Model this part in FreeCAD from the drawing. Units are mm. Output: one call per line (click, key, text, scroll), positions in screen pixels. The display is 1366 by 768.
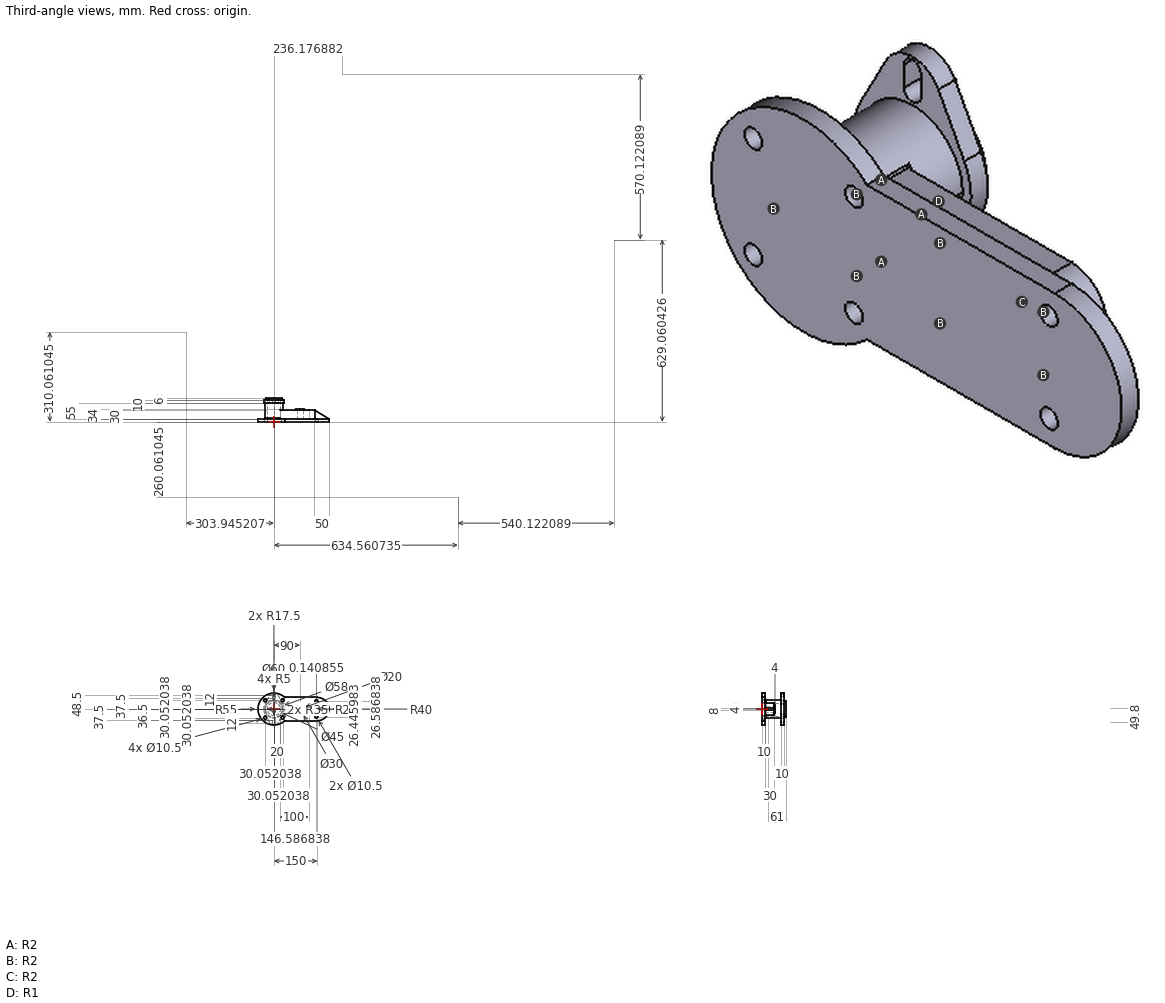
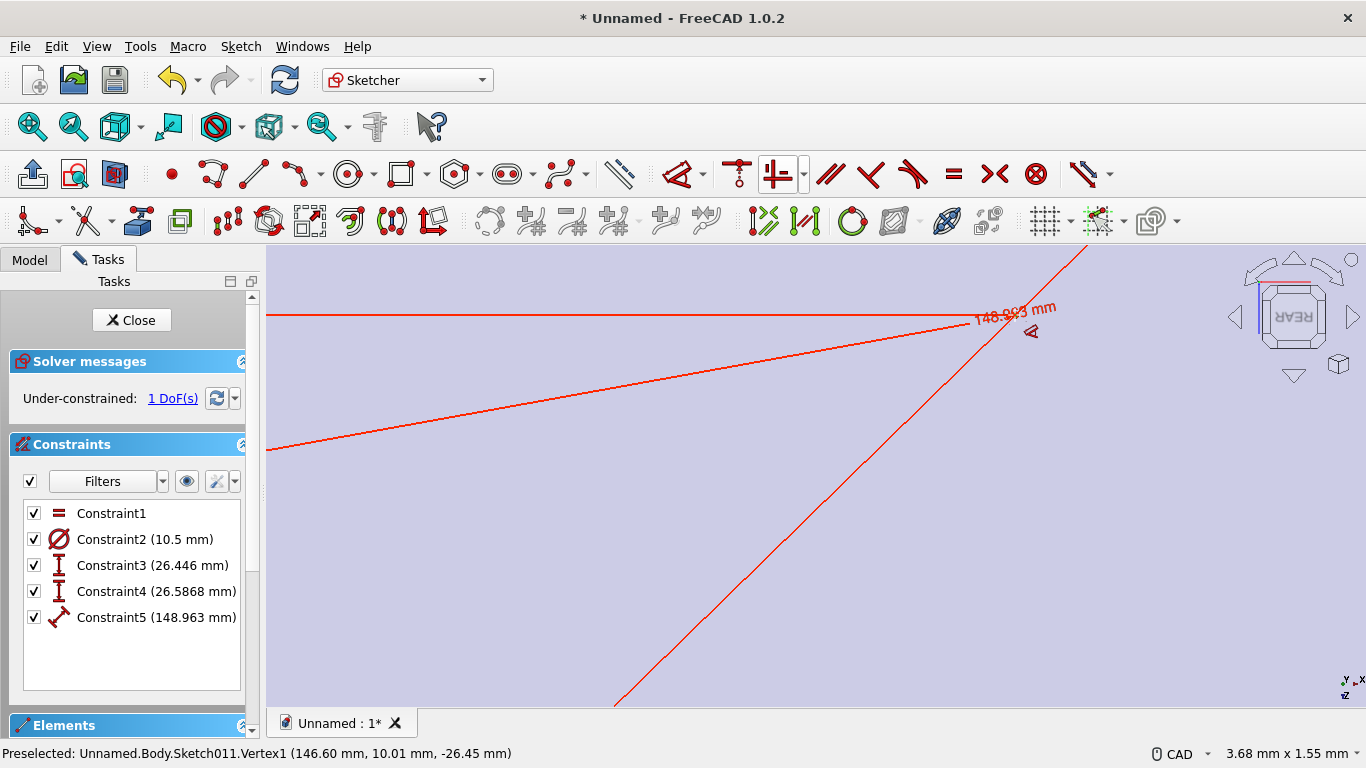
scroll(748, 476, down, 15)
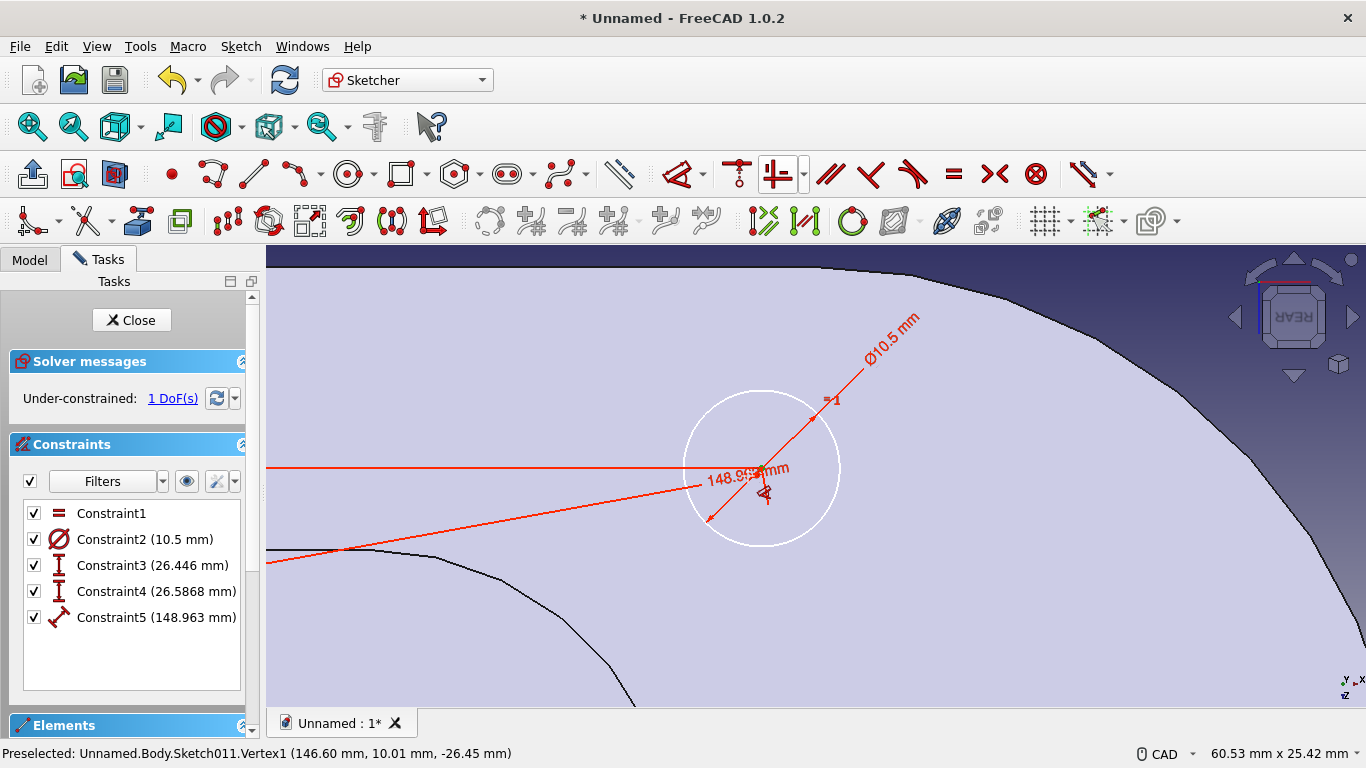
scroll(1195, 309, down, 6)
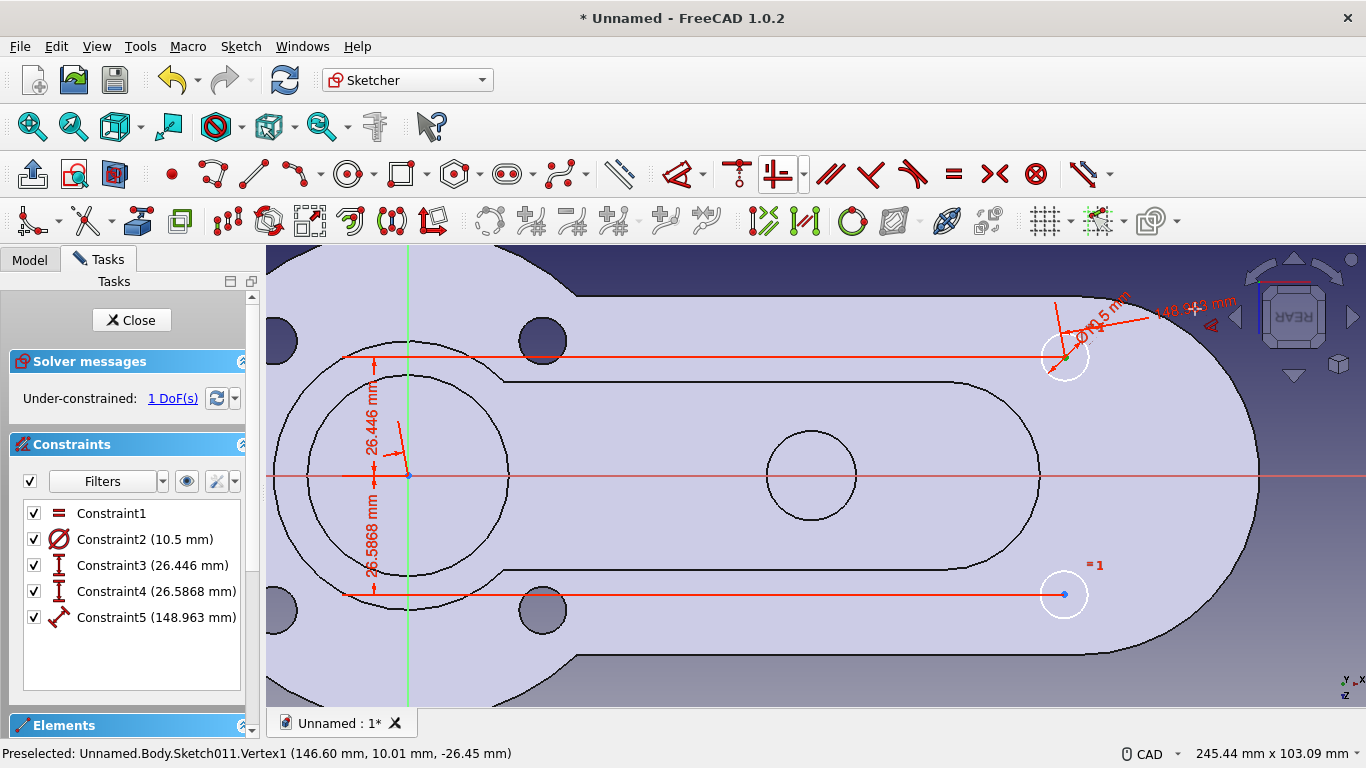
scroll(1064, 595, up, 21)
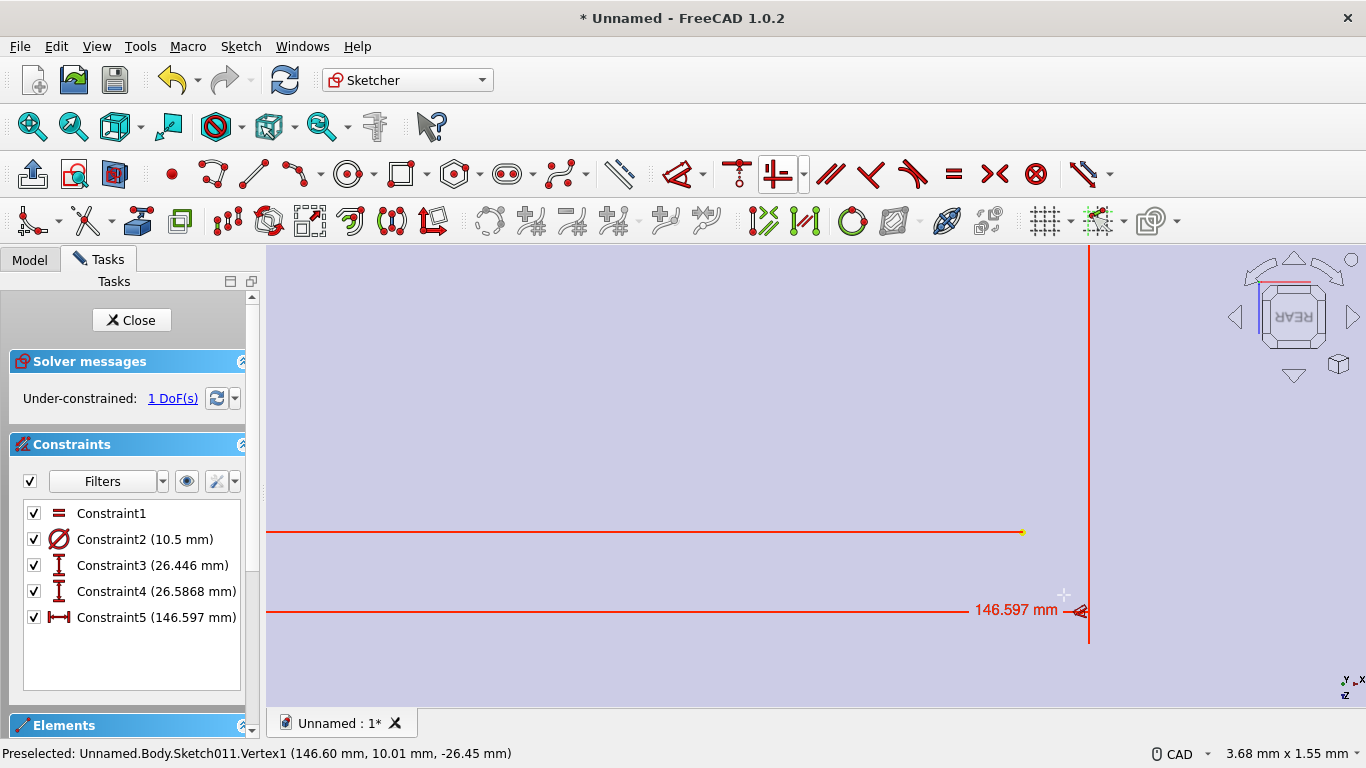
click(1022, 532)
click(1056, 566)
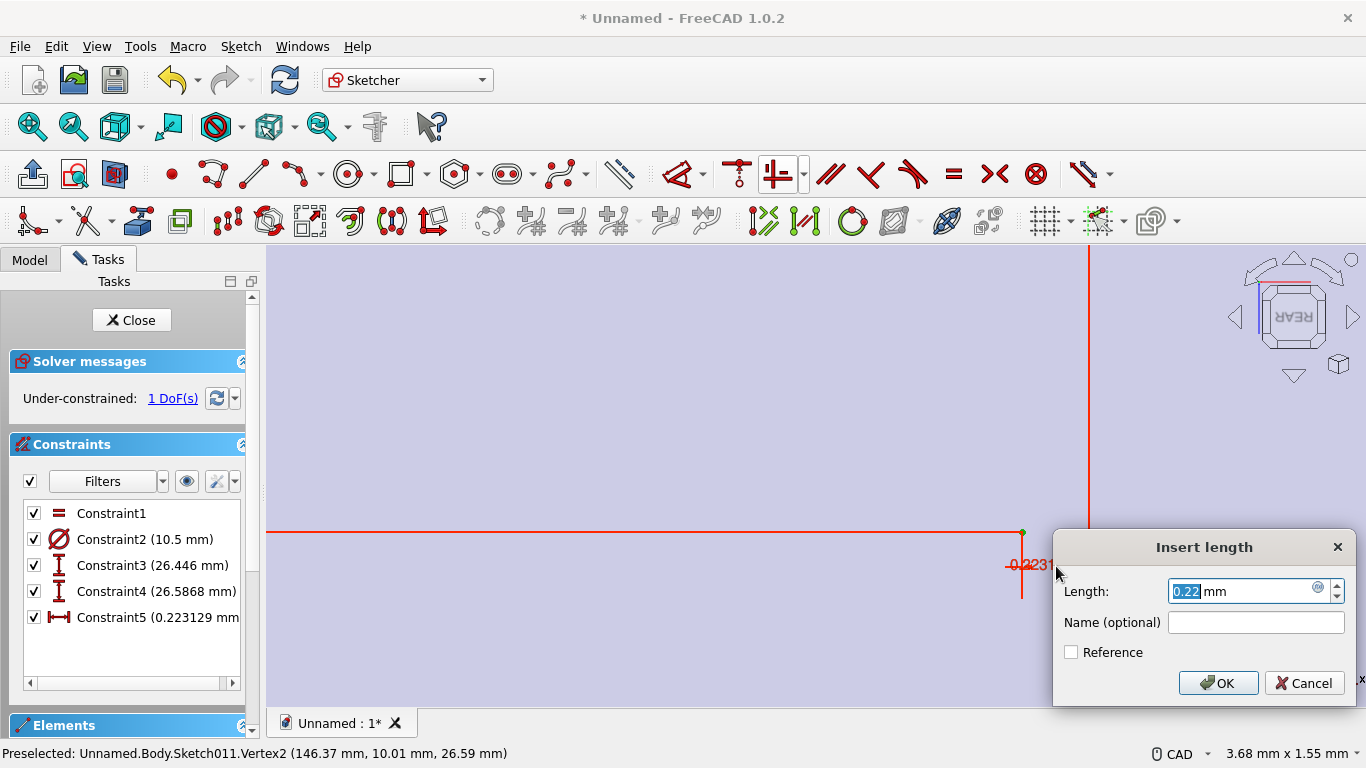
text(0.140855)
key(Return)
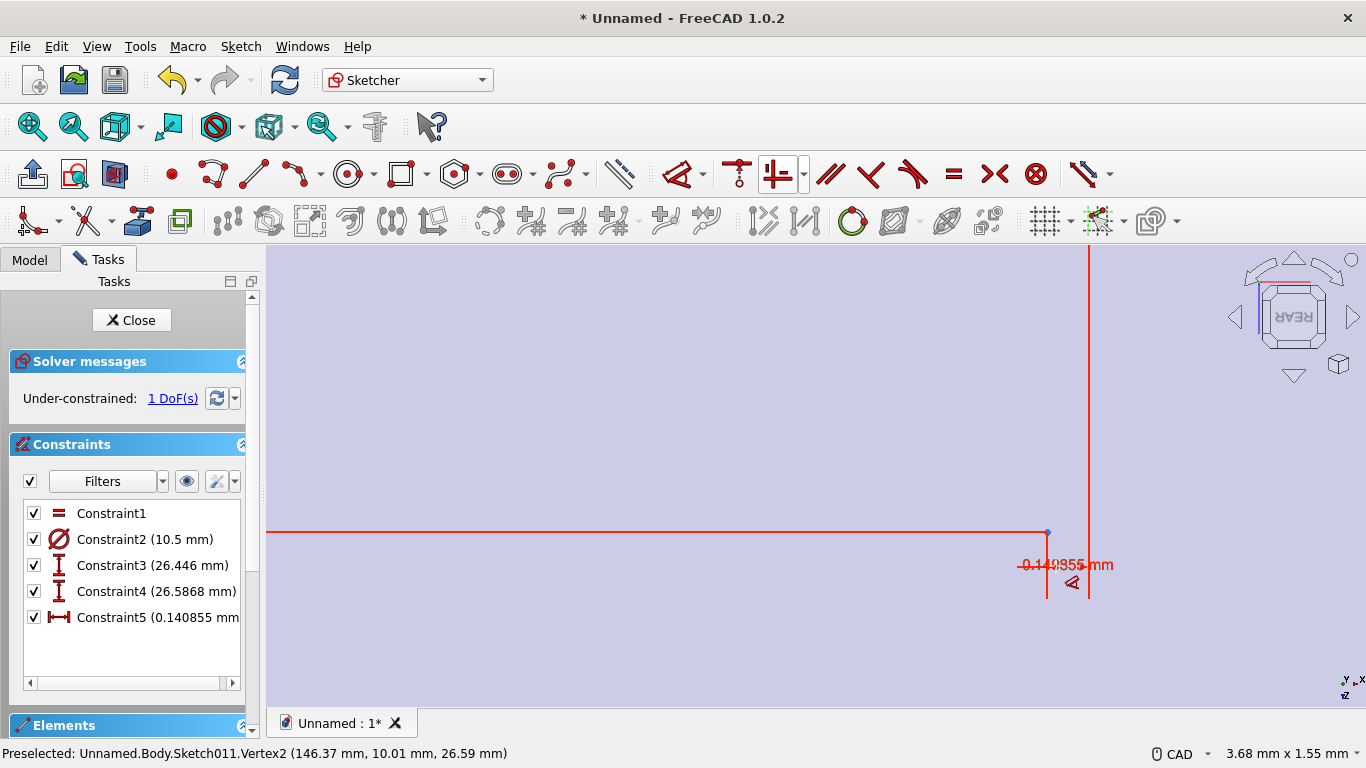
scroll(748, 476, down, 15)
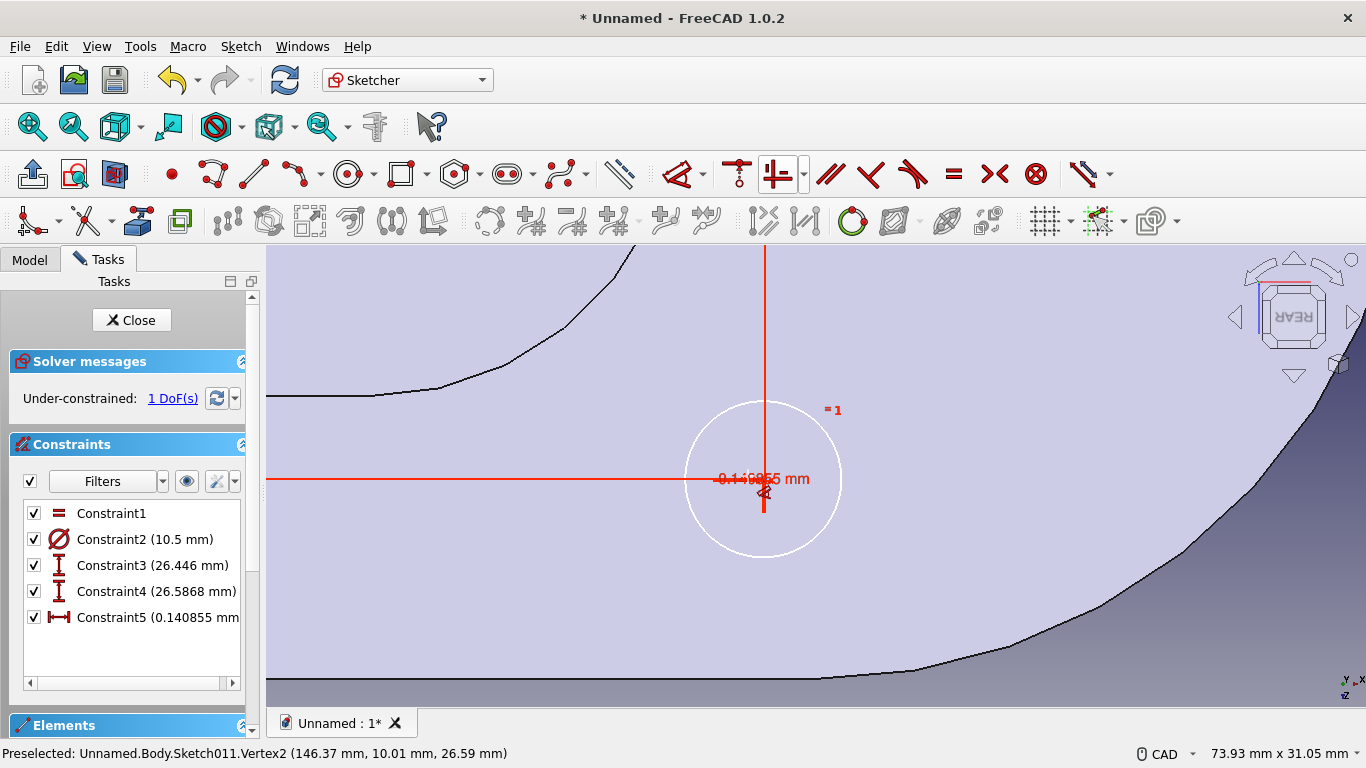
scroll(1193, 645, down, 6)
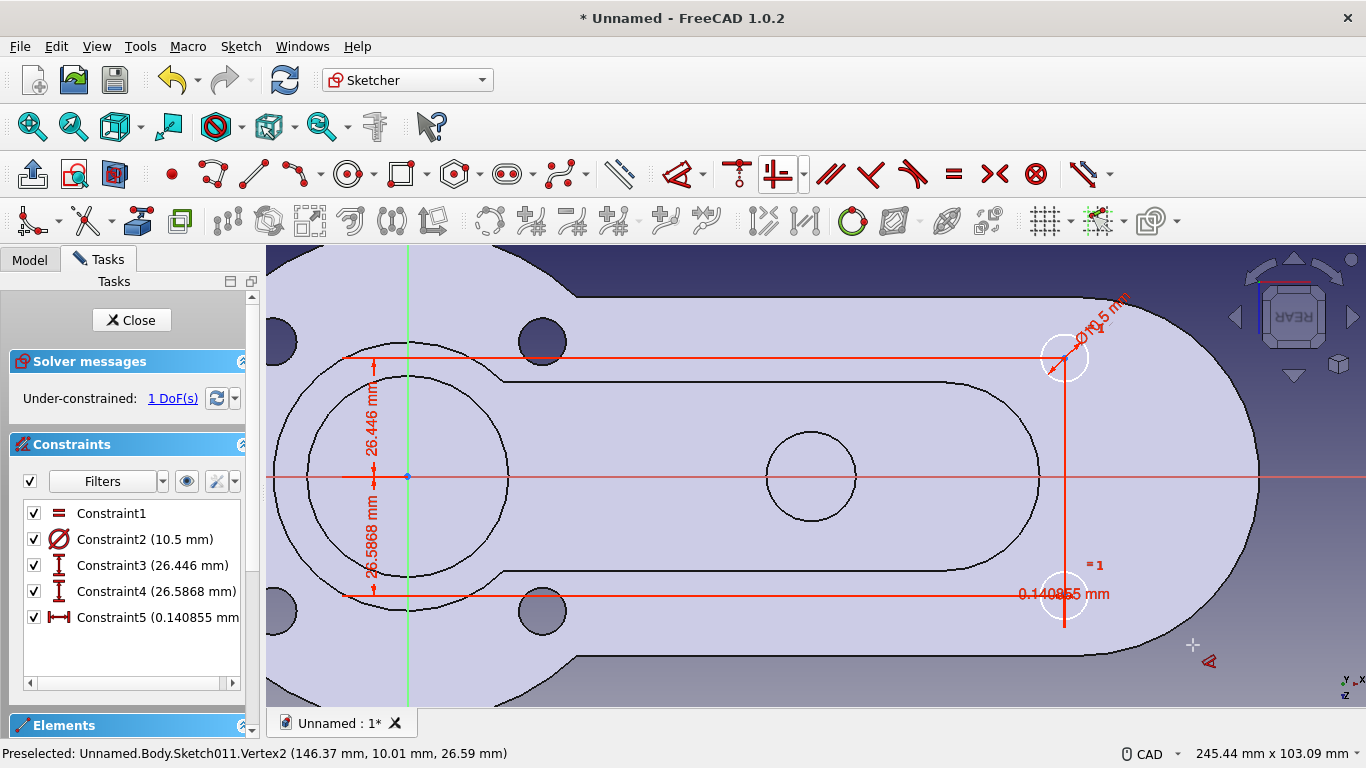
click(1065, 358)
click(736, 324)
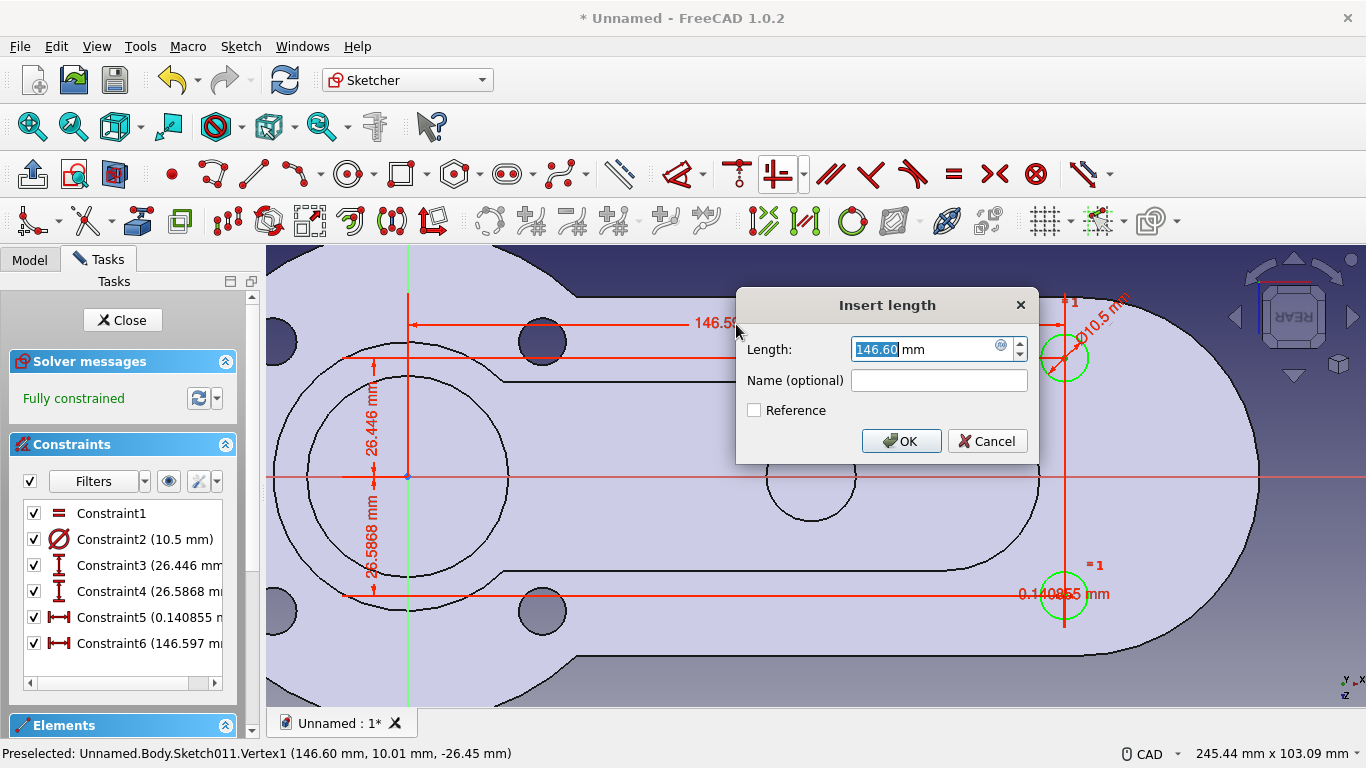
text(146.586838)
key(Return)
key(Escape)